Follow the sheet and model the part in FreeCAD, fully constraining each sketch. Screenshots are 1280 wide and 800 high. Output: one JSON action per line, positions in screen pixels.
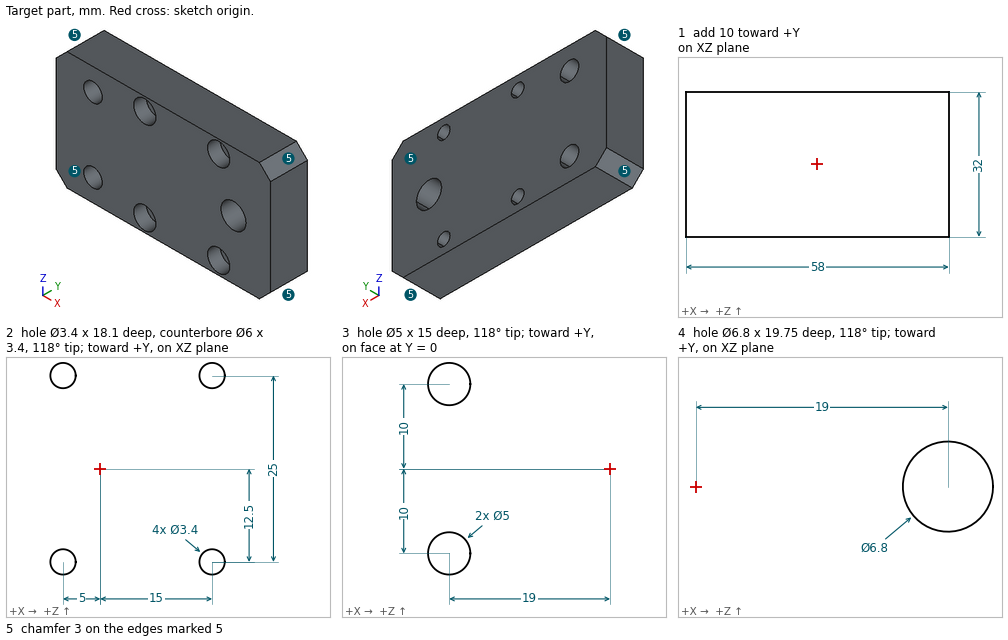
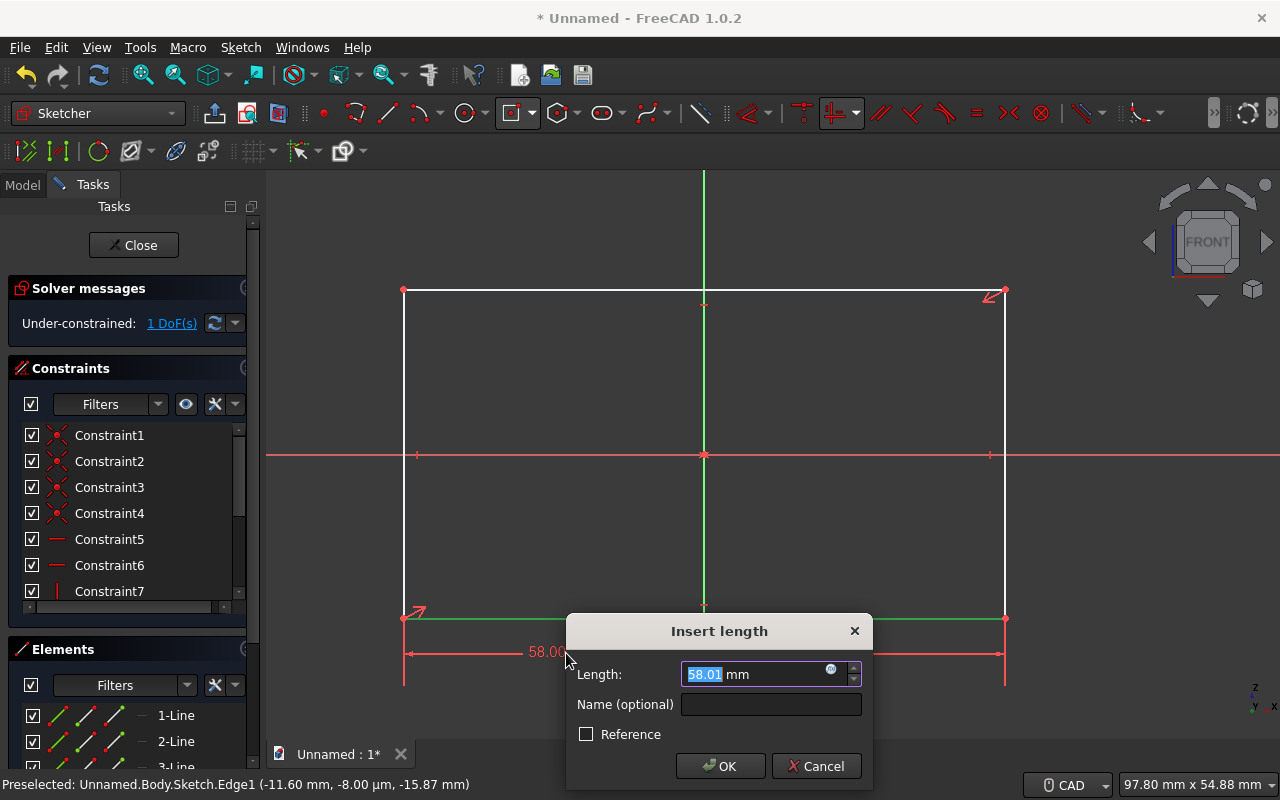
{"action": "type", "text": "58"}
{"action": "key", "text": "Return"}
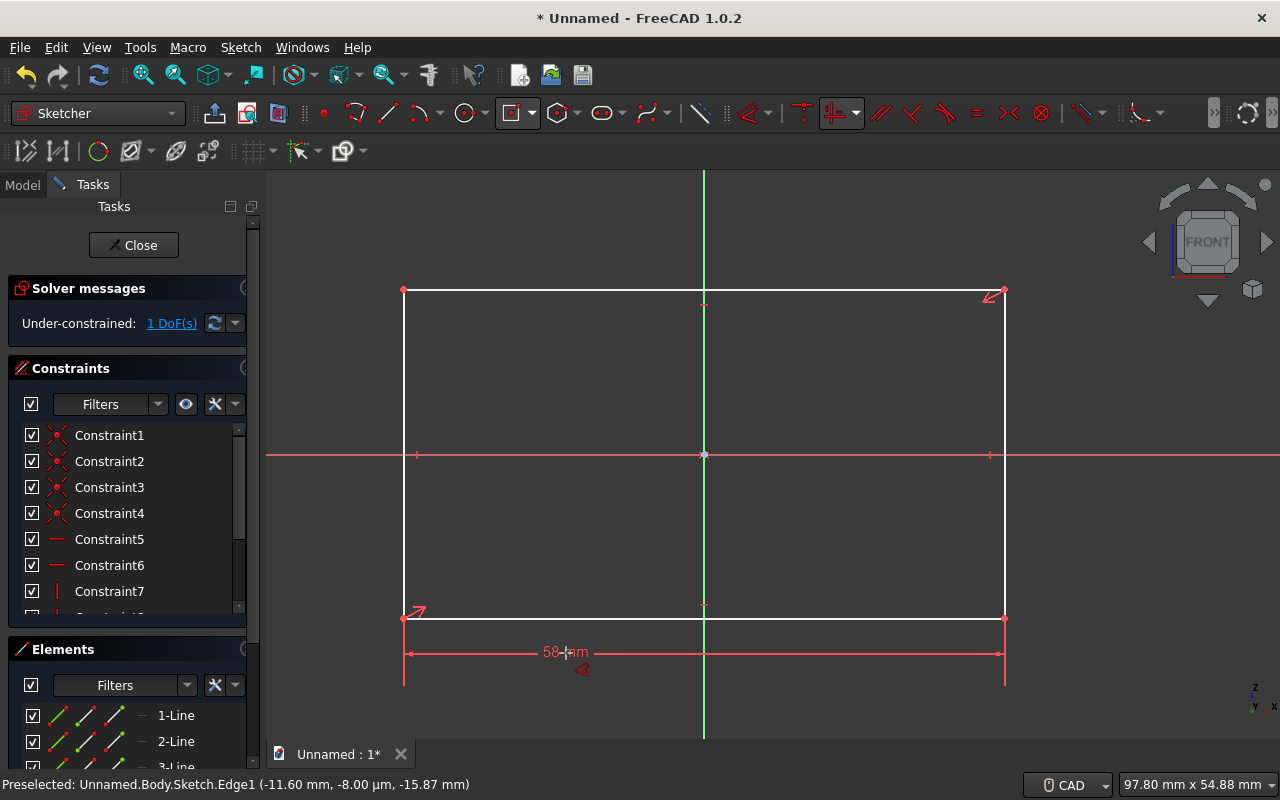
{"action": "left_click", "coordinate": [1005, 520]}
{"action": "left_click", "coordinate": [1039, 379]}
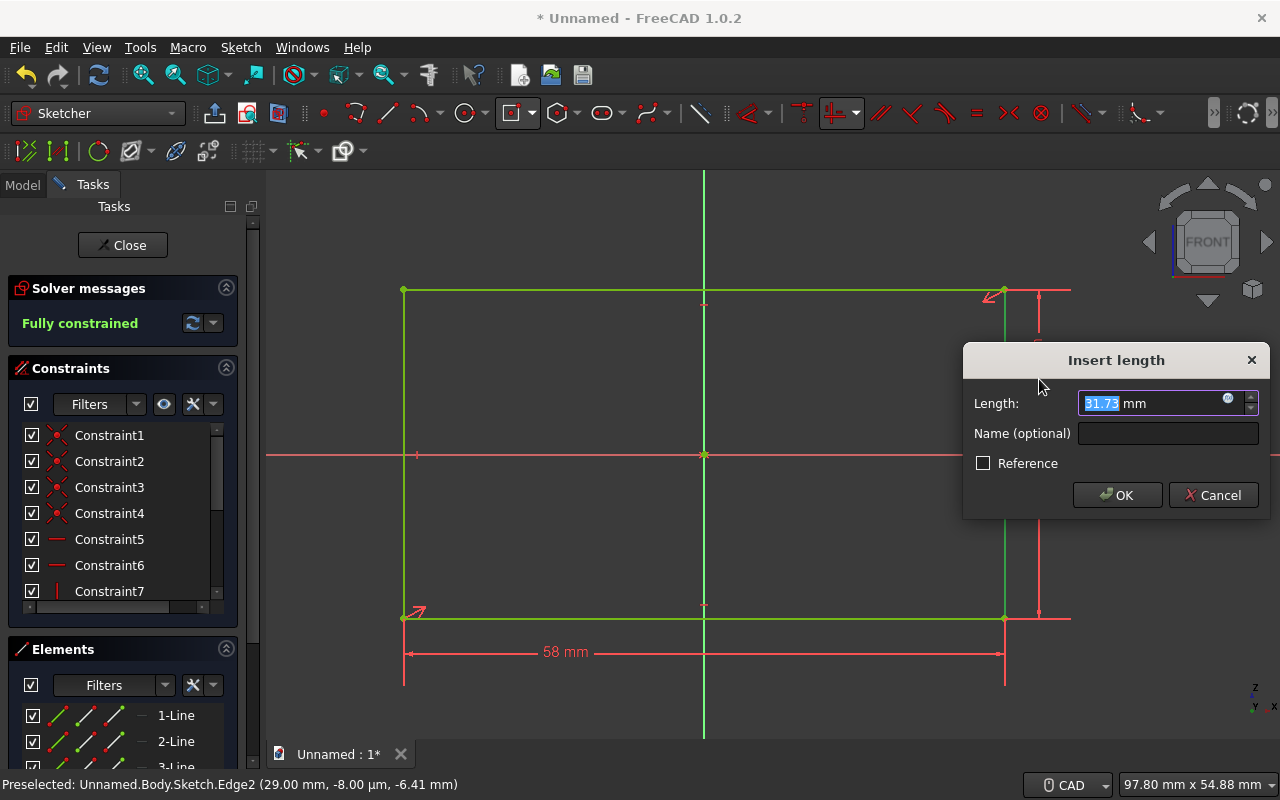
{"action": "type", "text": "32"}
{"action": "key", "text": "Return"}
{"action": "key", "text": "Escape"}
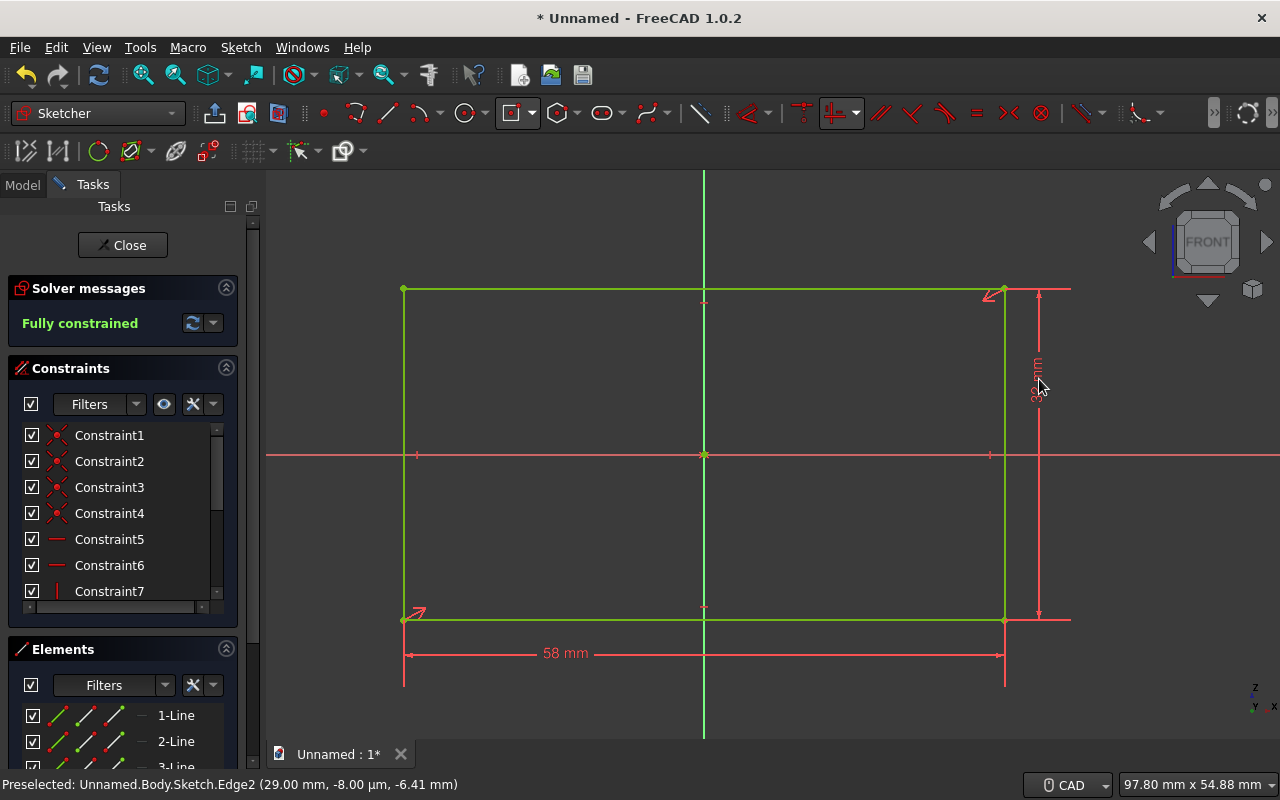
{"action": "left_click", "coordinate": [123, 245]}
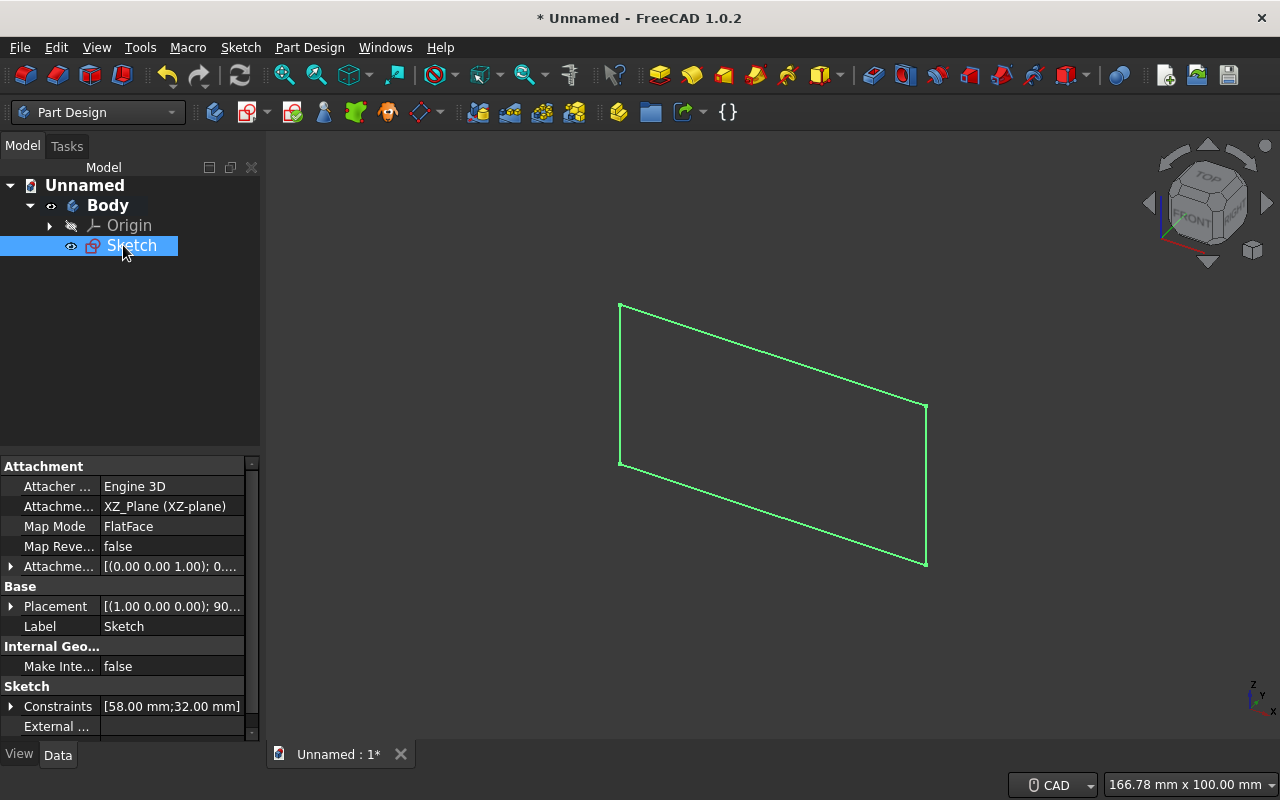
{"action": "left_click", "coordinate": [660, 76]}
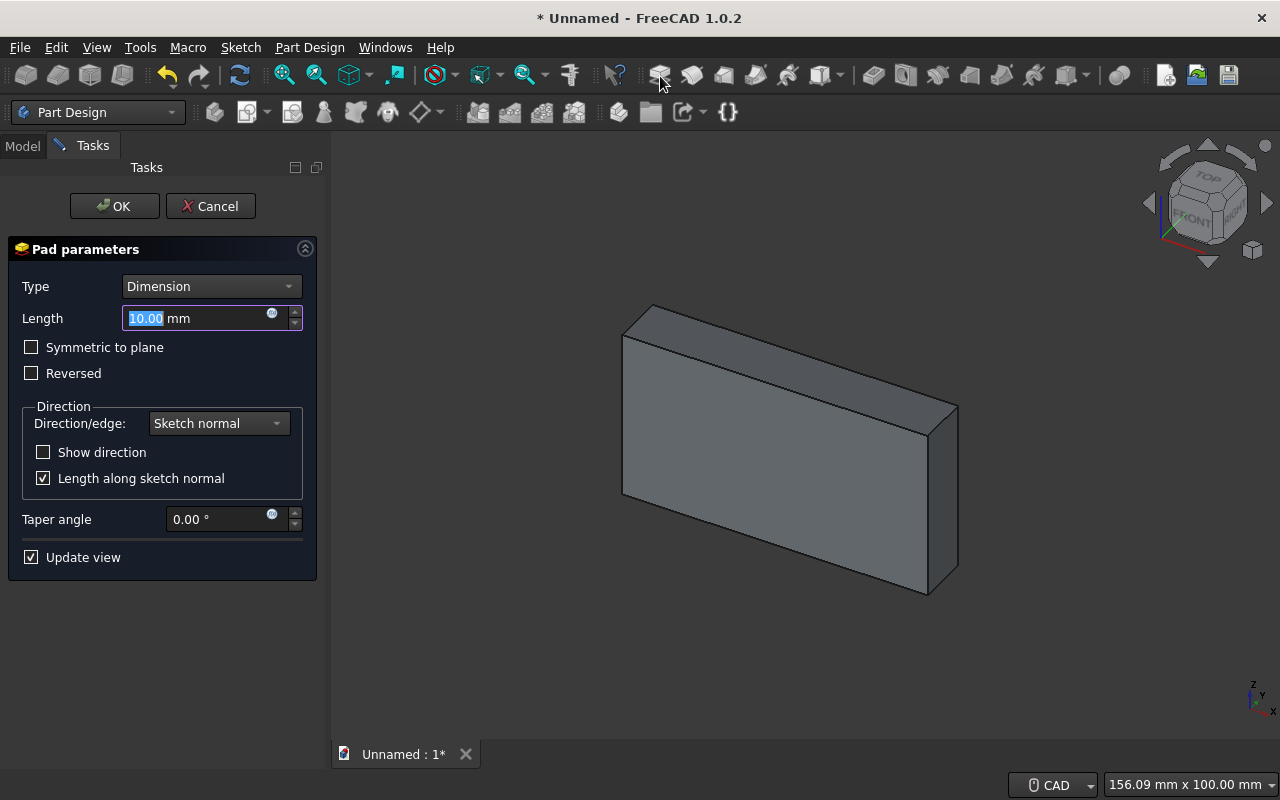
{"action": "type", "text": "10"}
{"action": "key", "text": "Tab"}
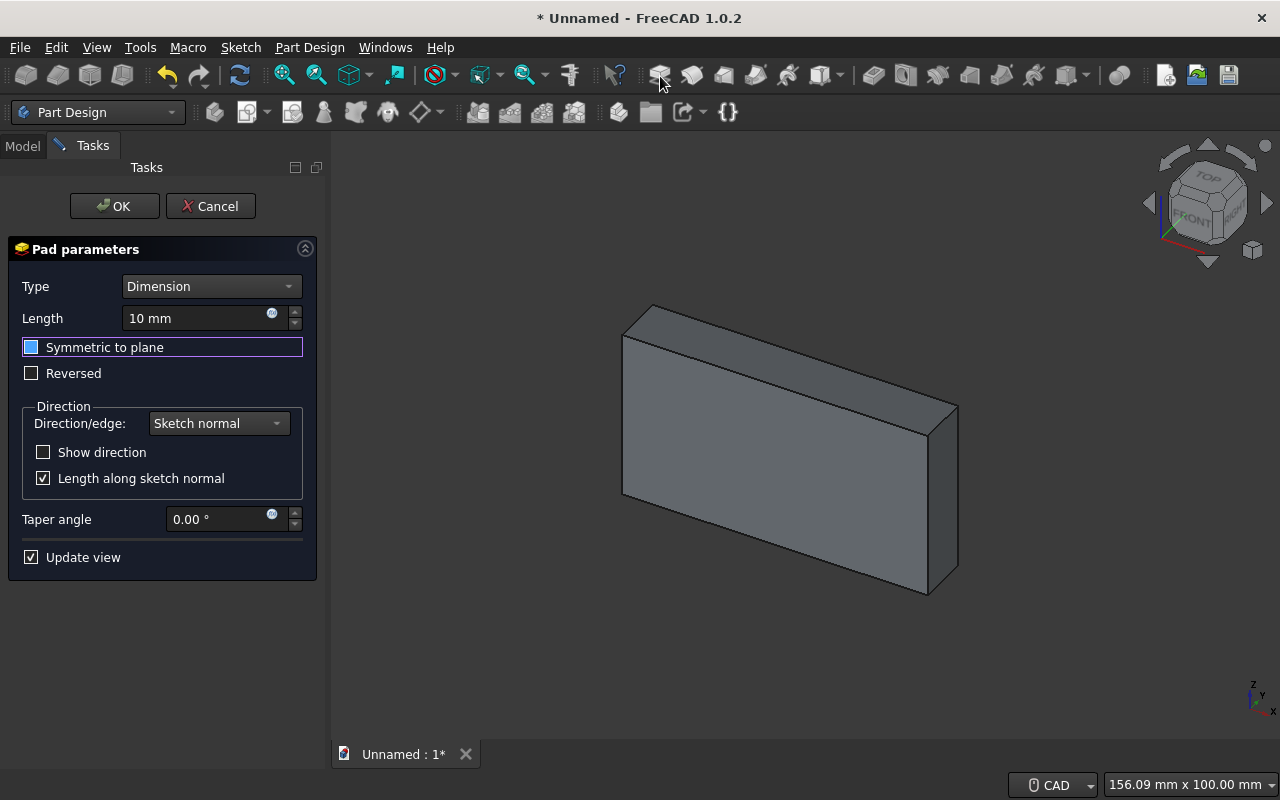
{"action": "left_click", "coordinate": [30, 373]}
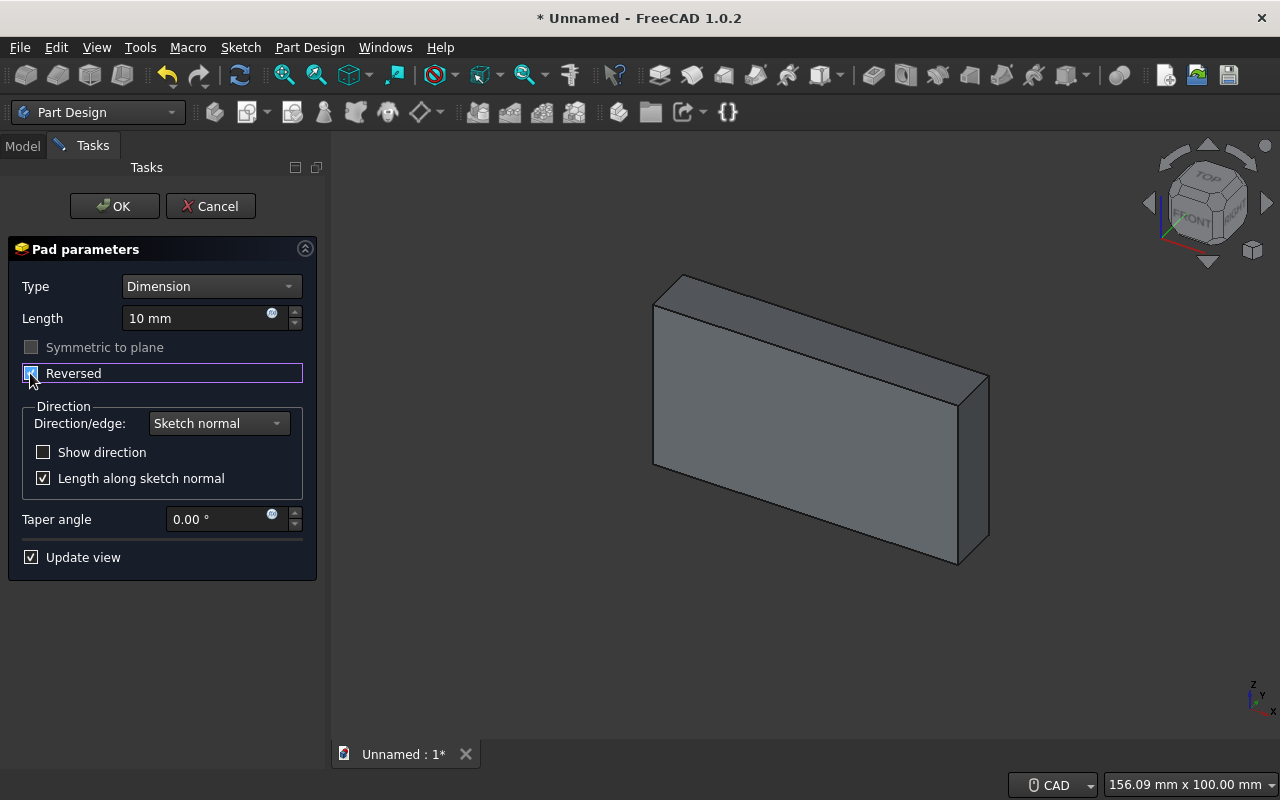
{"action": "left_click", "coordinate": [115, 206]}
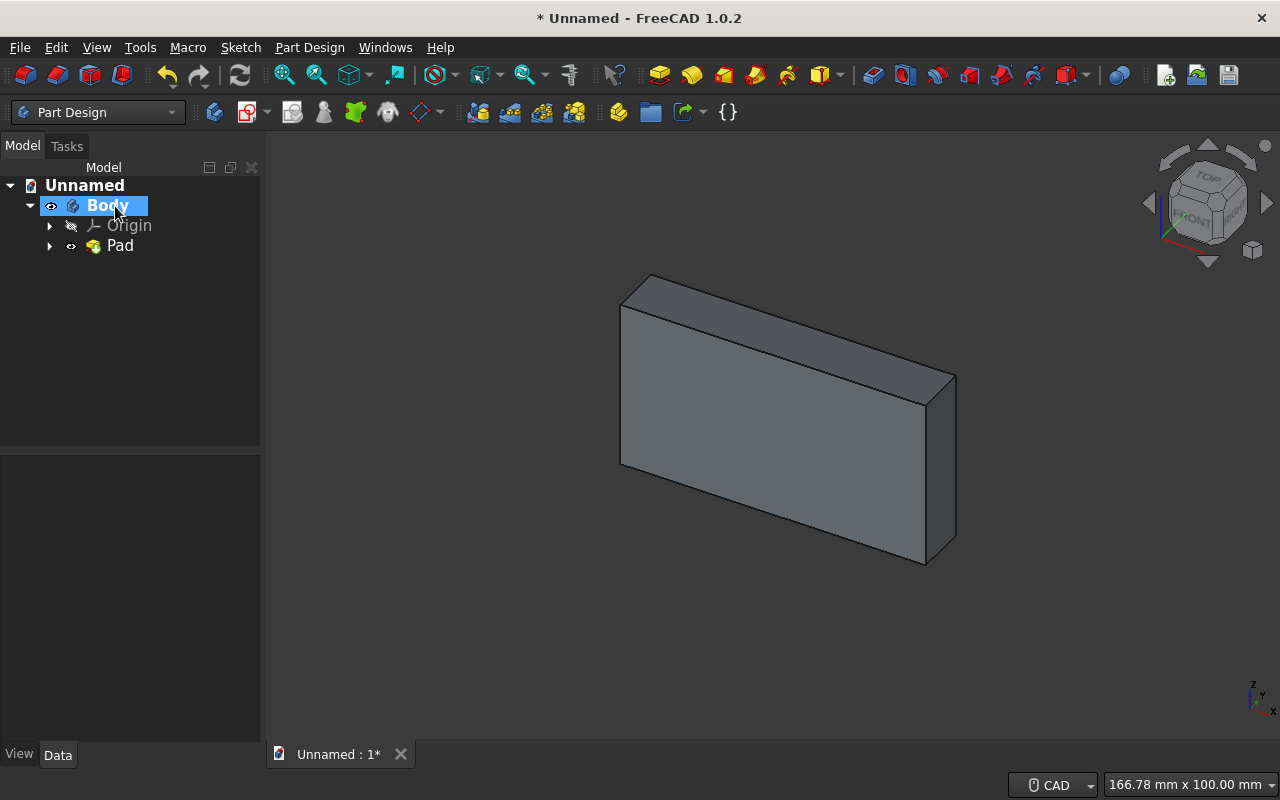
{"action": "left_click", "coordinate": [248, 112]}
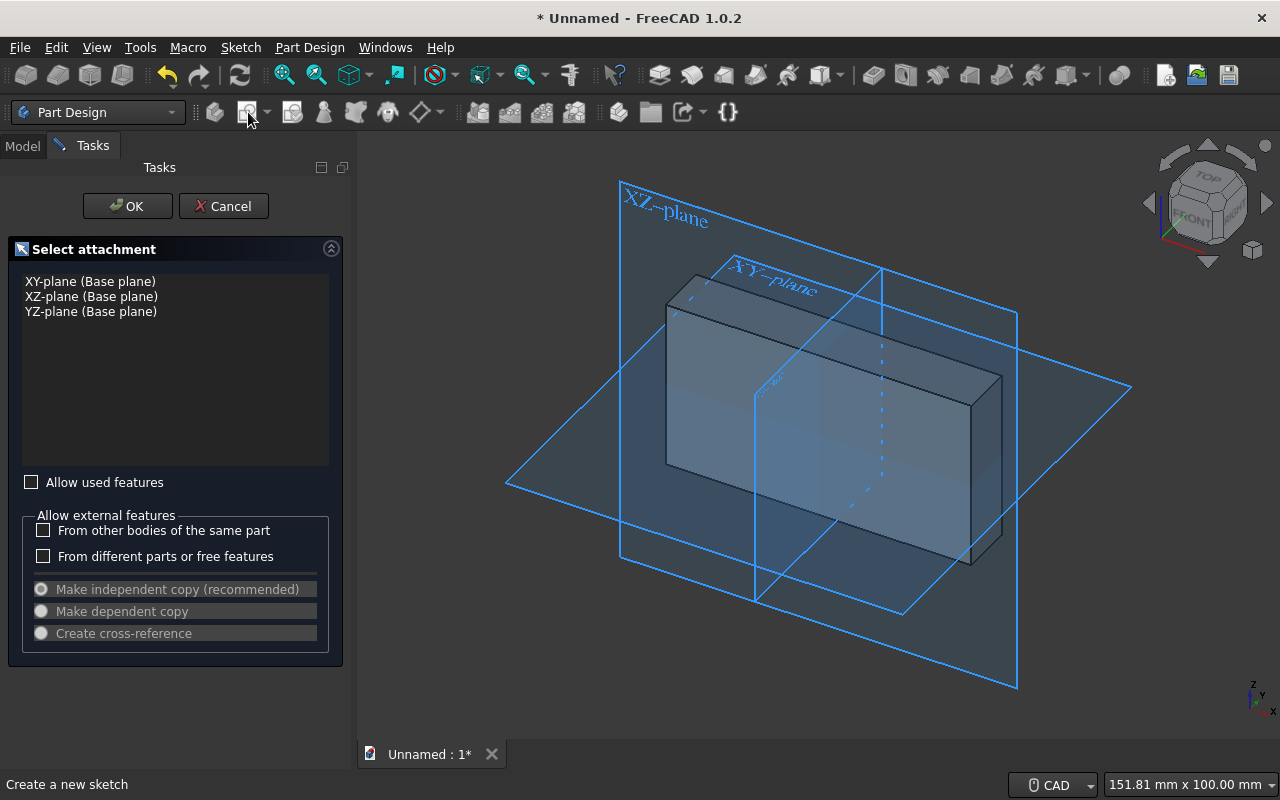
{"action": "left_click", "coordinate": [82, 296]}